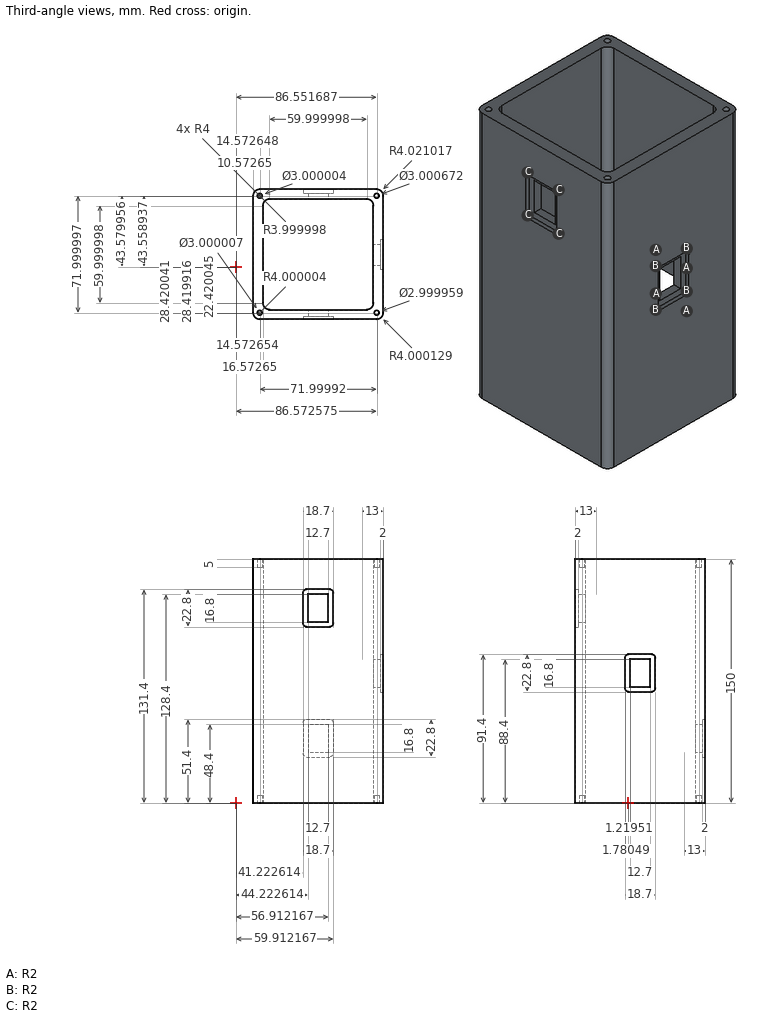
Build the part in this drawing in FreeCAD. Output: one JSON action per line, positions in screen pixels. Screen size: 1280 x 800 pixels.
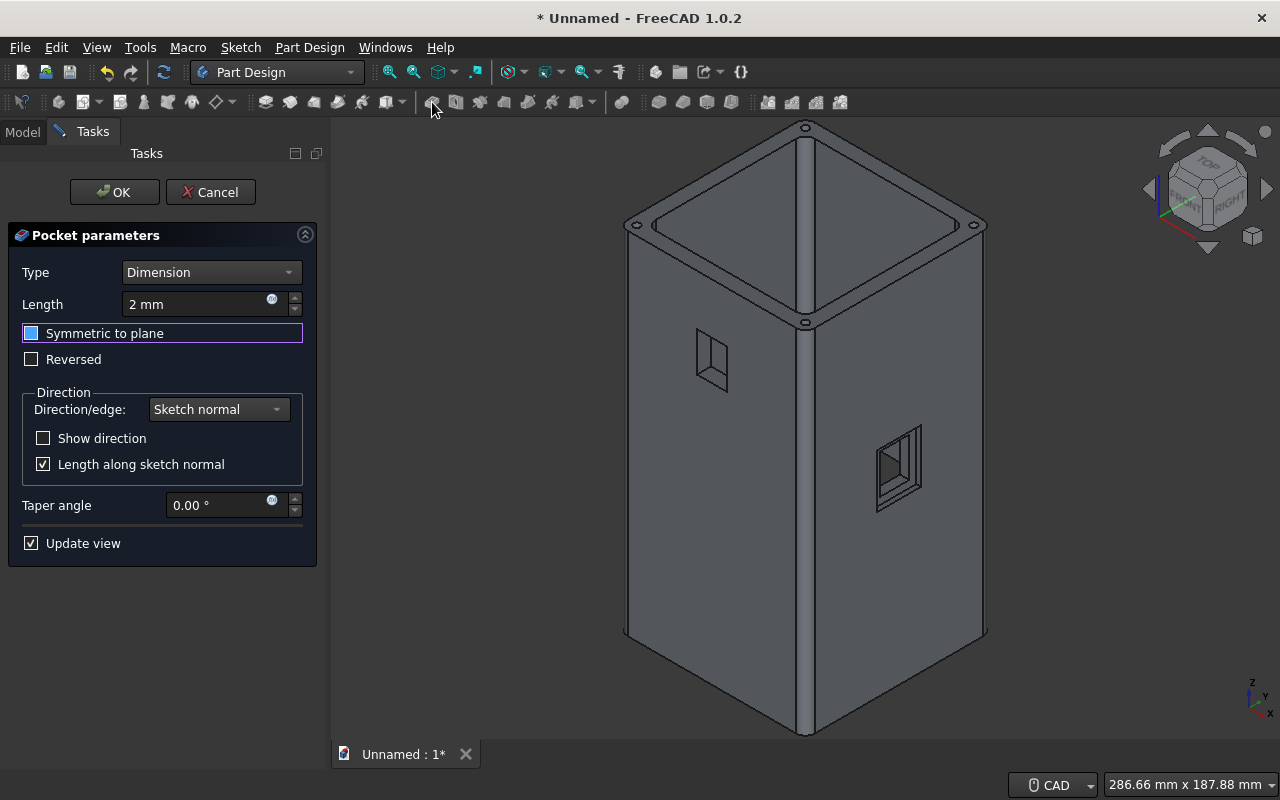
{"action": "left_click", "coordinate": [115, 192]}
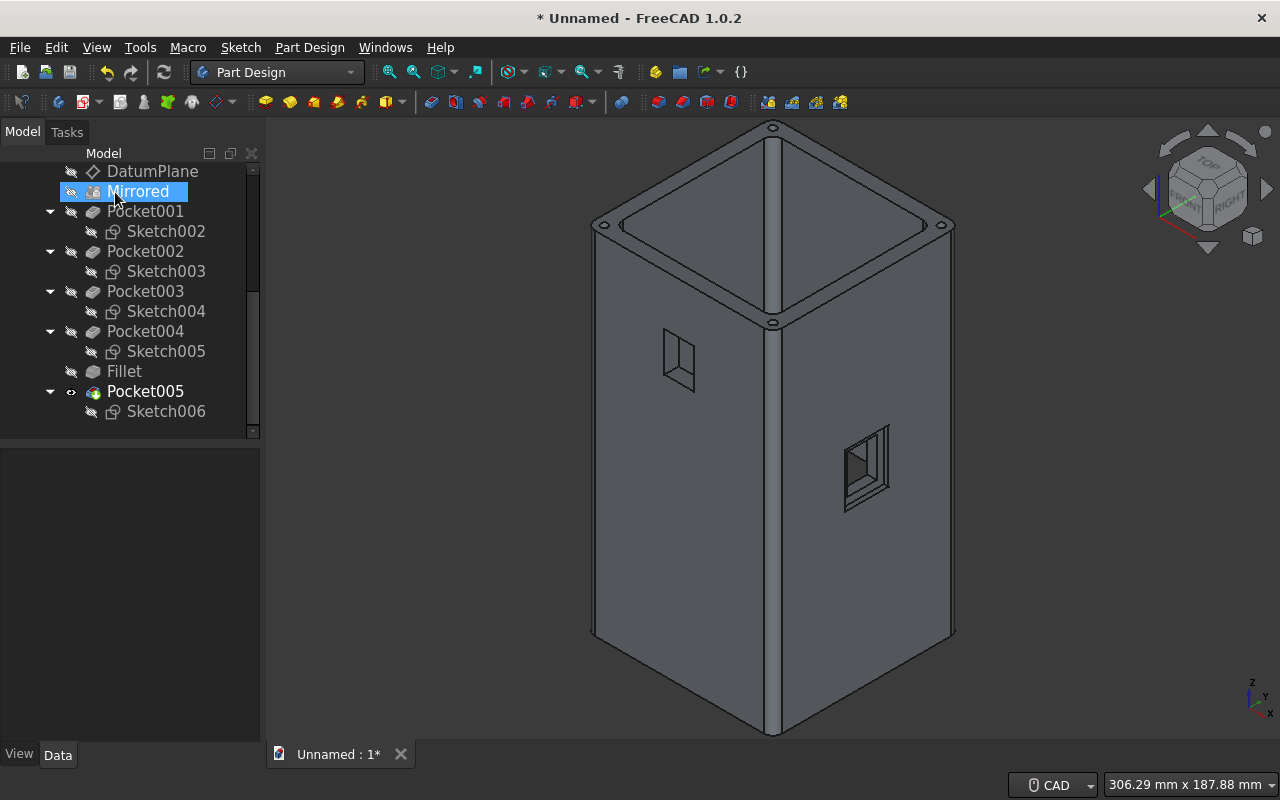
{"action": "key", "text": "v f"}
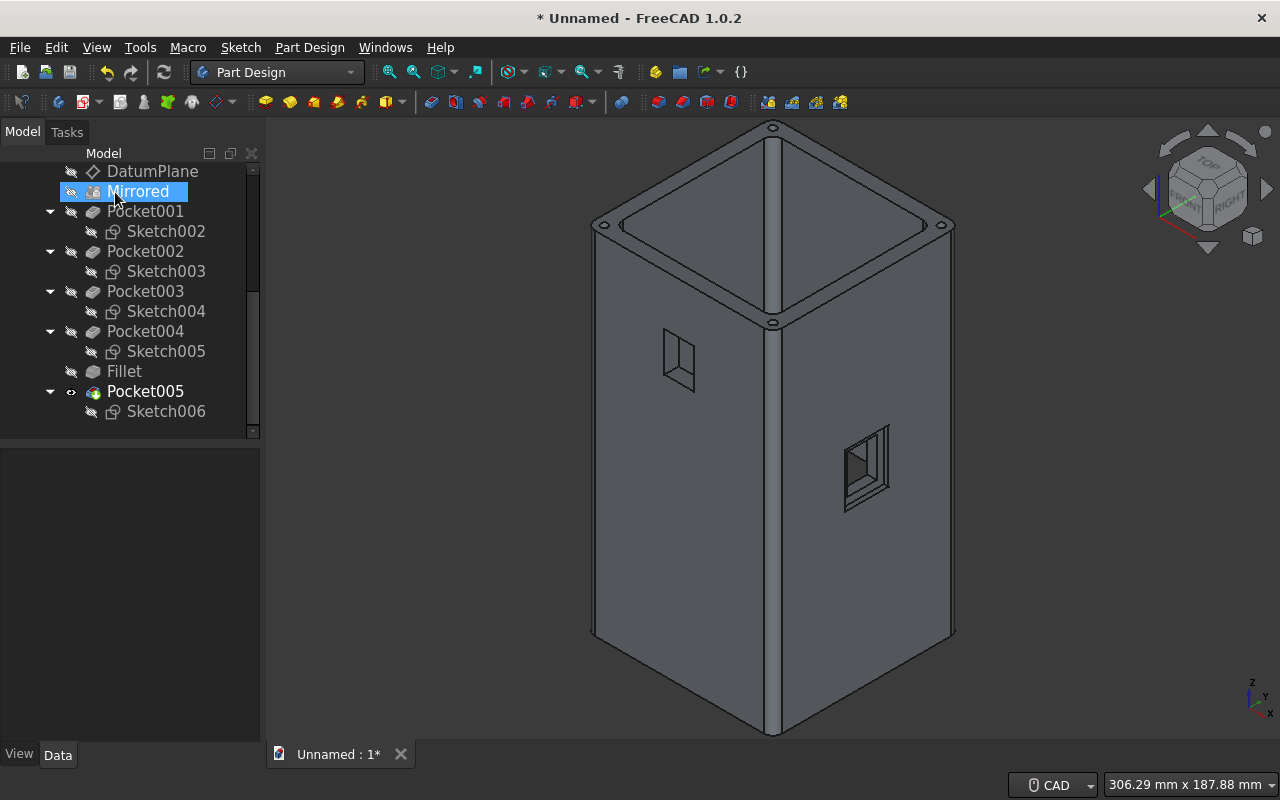
{"action": "scroll", "coordinate": [886, 423], "scroll_direction": "up", "scroll_amount": 9}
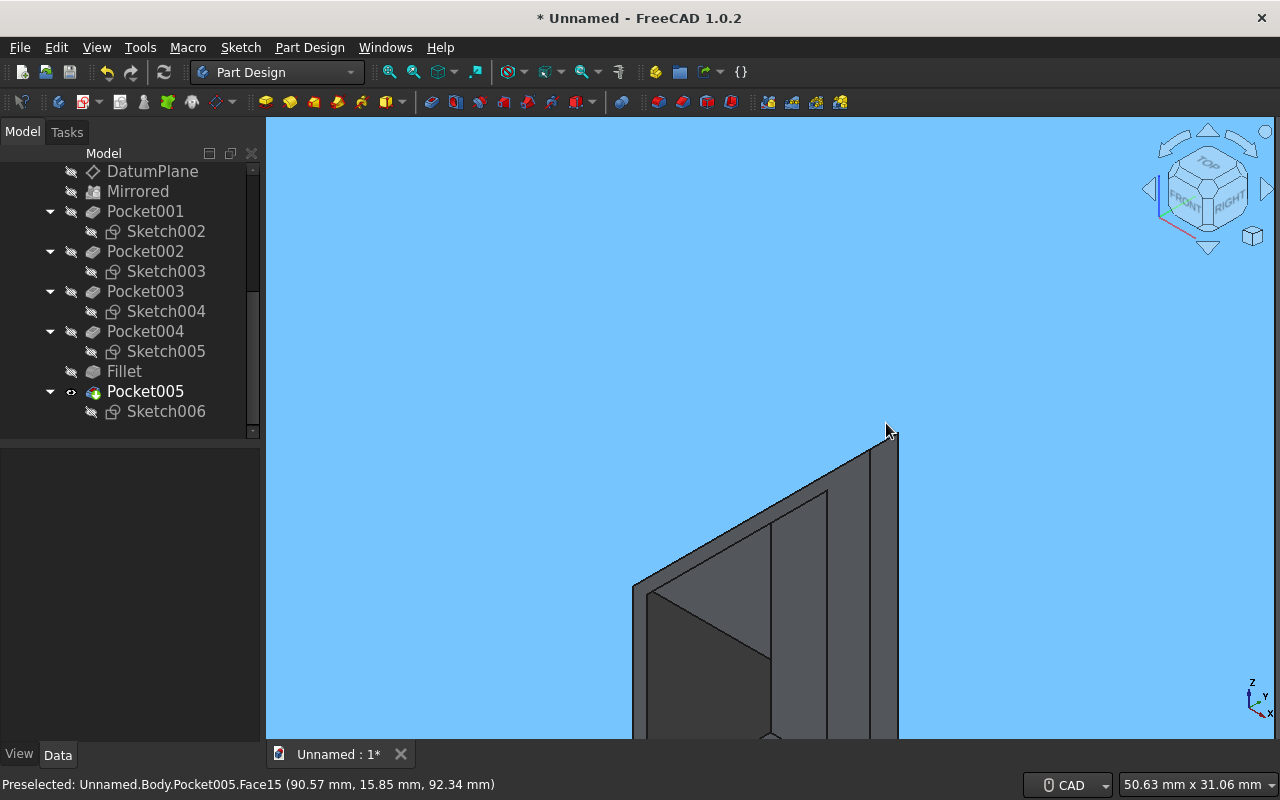
{"action": "left_click", "coordinate": [390, 72]}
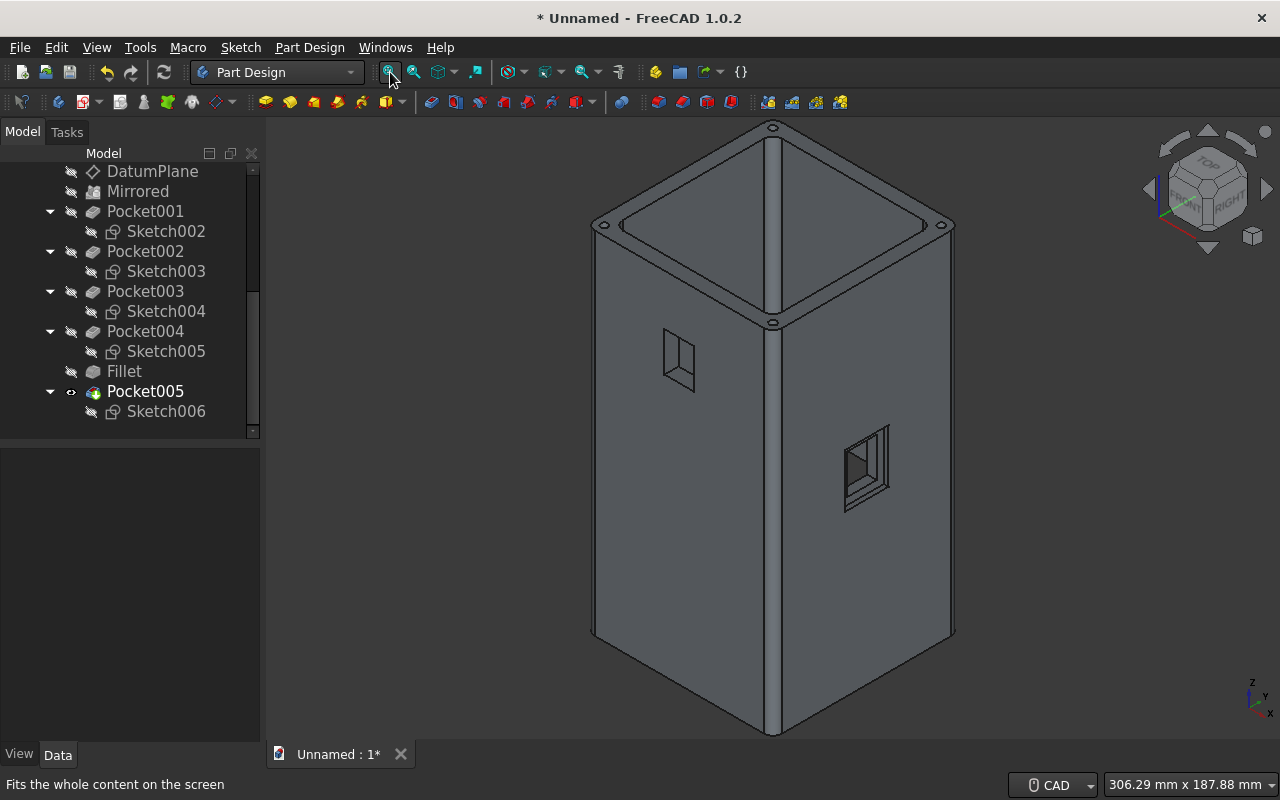
{"action": "key", "text": "2"}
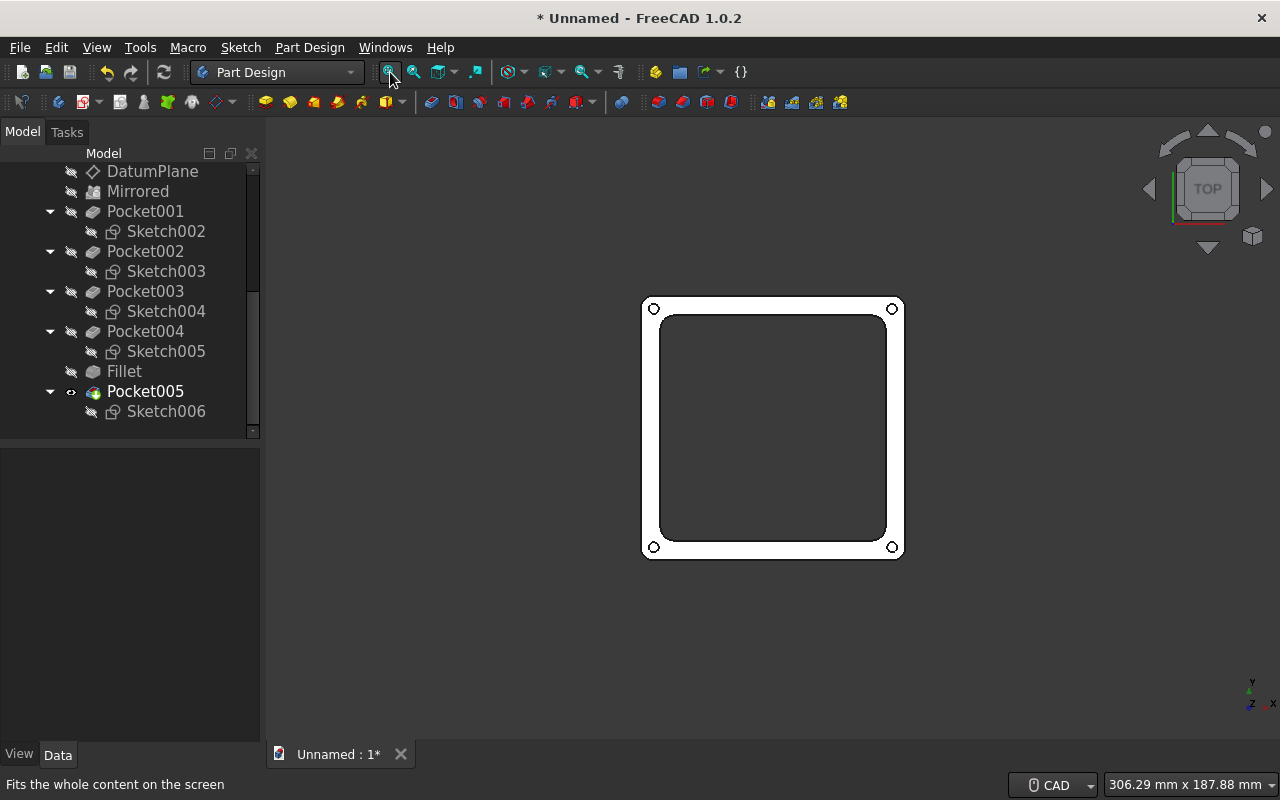
{"action": "left_click", "coordinate": [390, 72]}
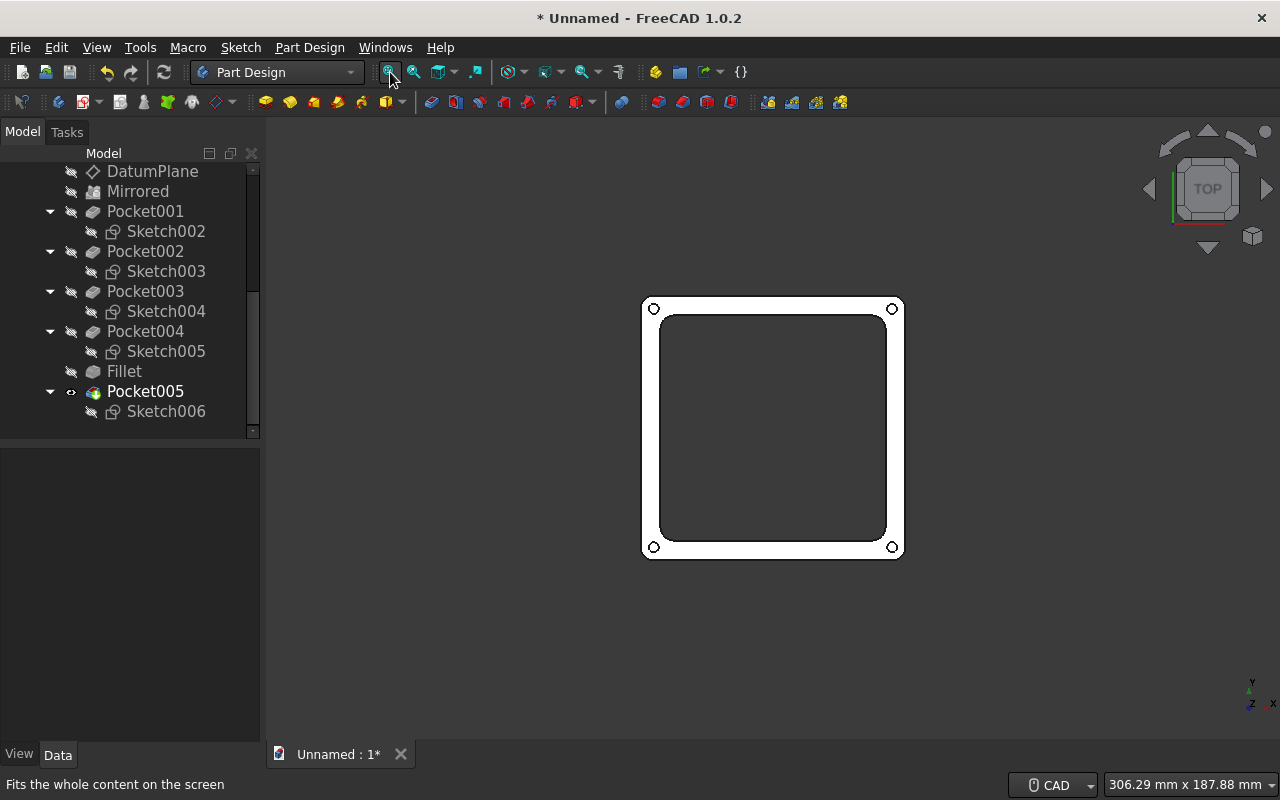
{"action": "scroll", "coordinate": [902, 396], "scroll_direction": "up", "scroll_amount": 9}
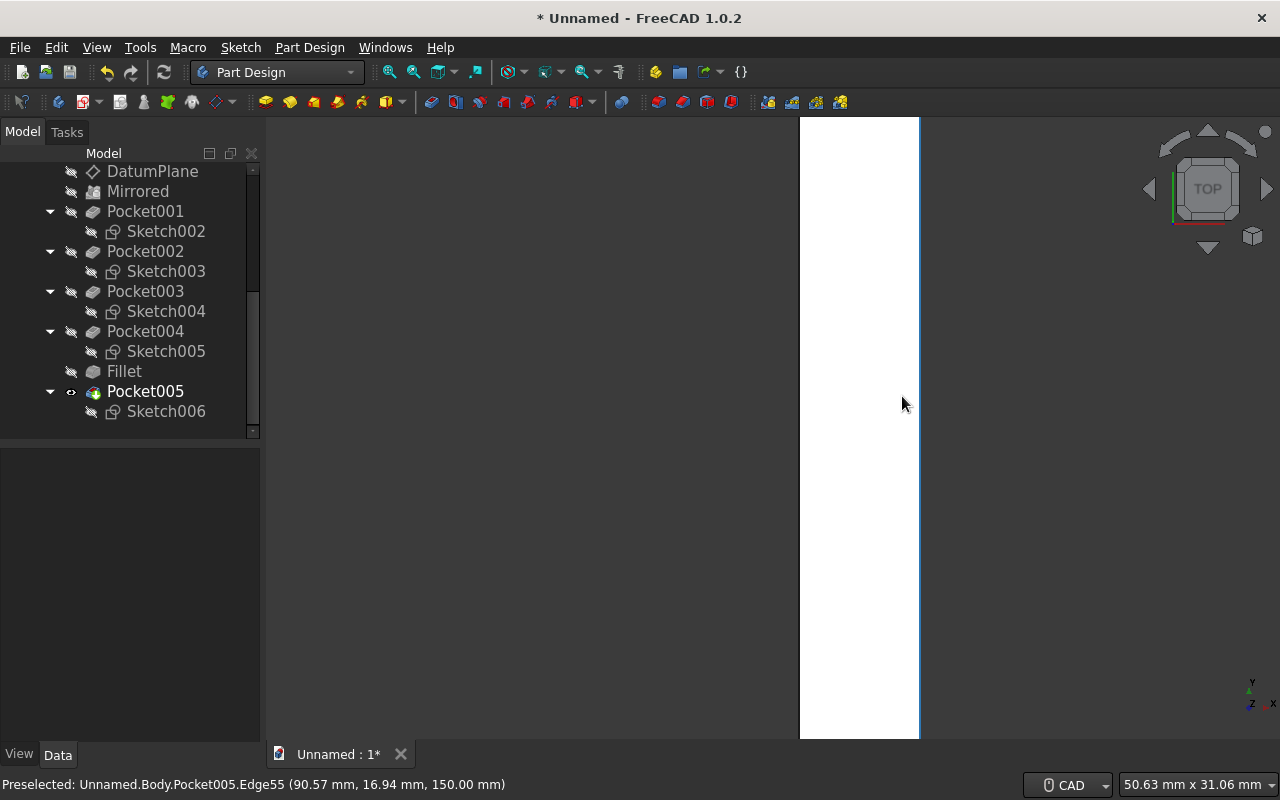
{"action": "left_click", "coordinate": [390, 72]}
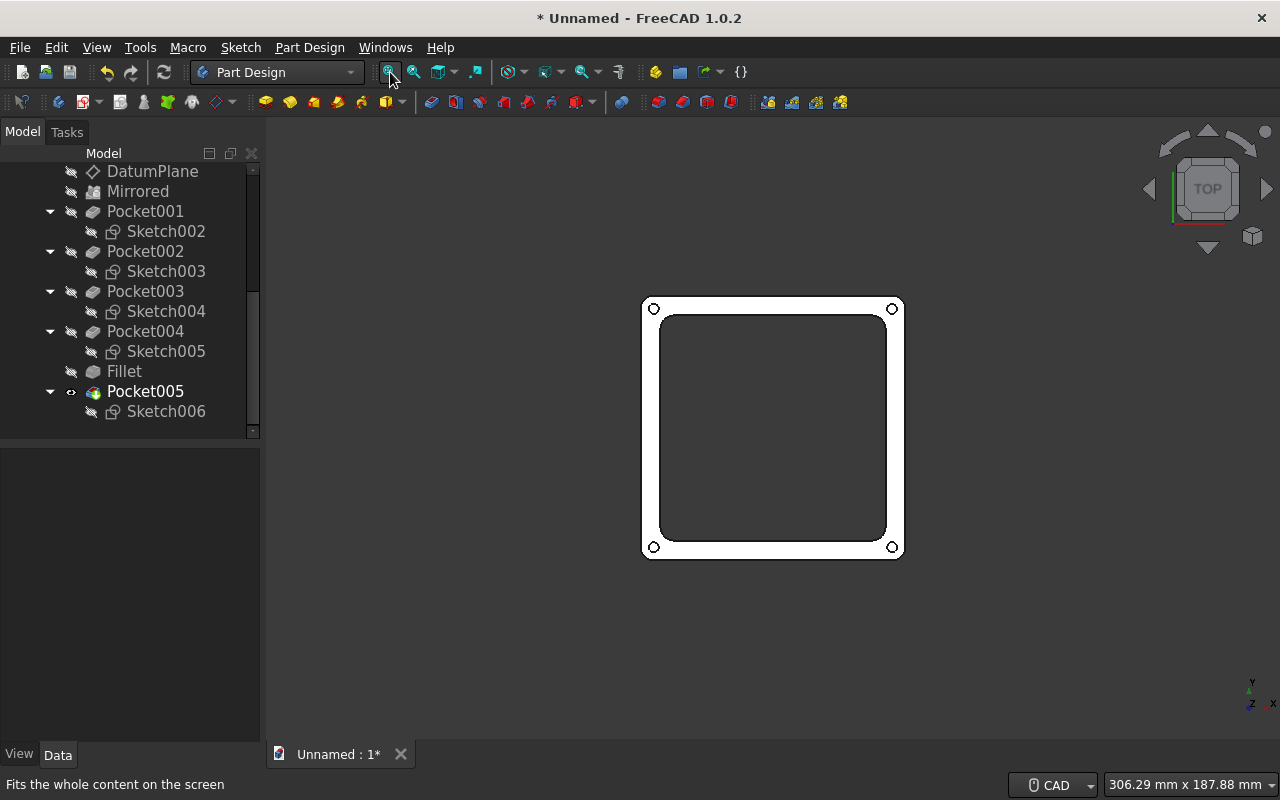
{"action": "key", "text": "0"}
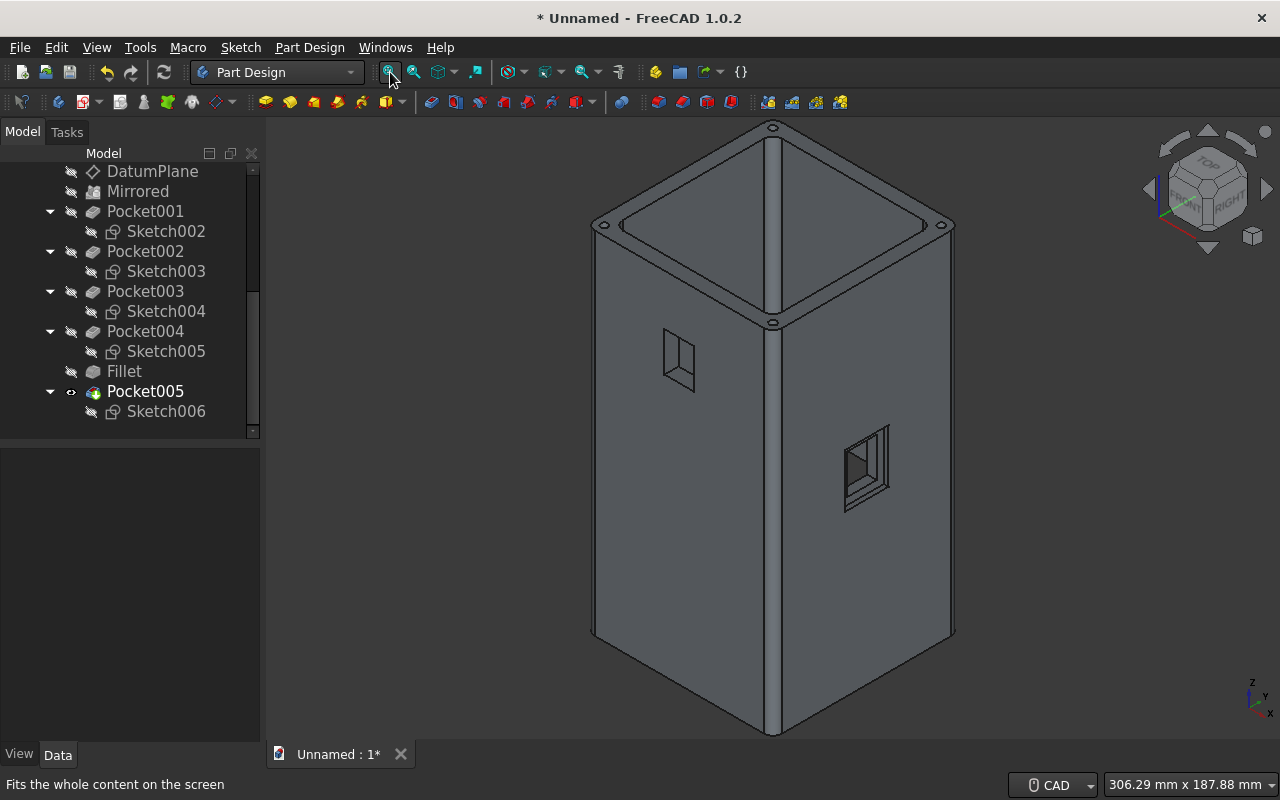
{"action": "key", "text": "v f"}